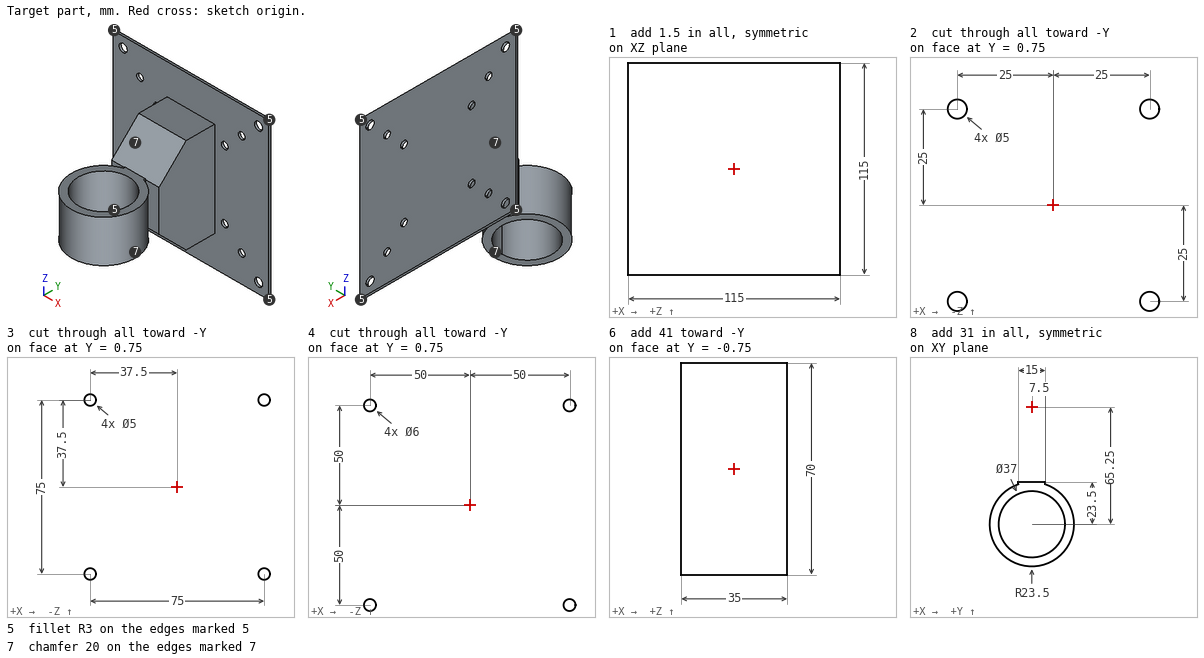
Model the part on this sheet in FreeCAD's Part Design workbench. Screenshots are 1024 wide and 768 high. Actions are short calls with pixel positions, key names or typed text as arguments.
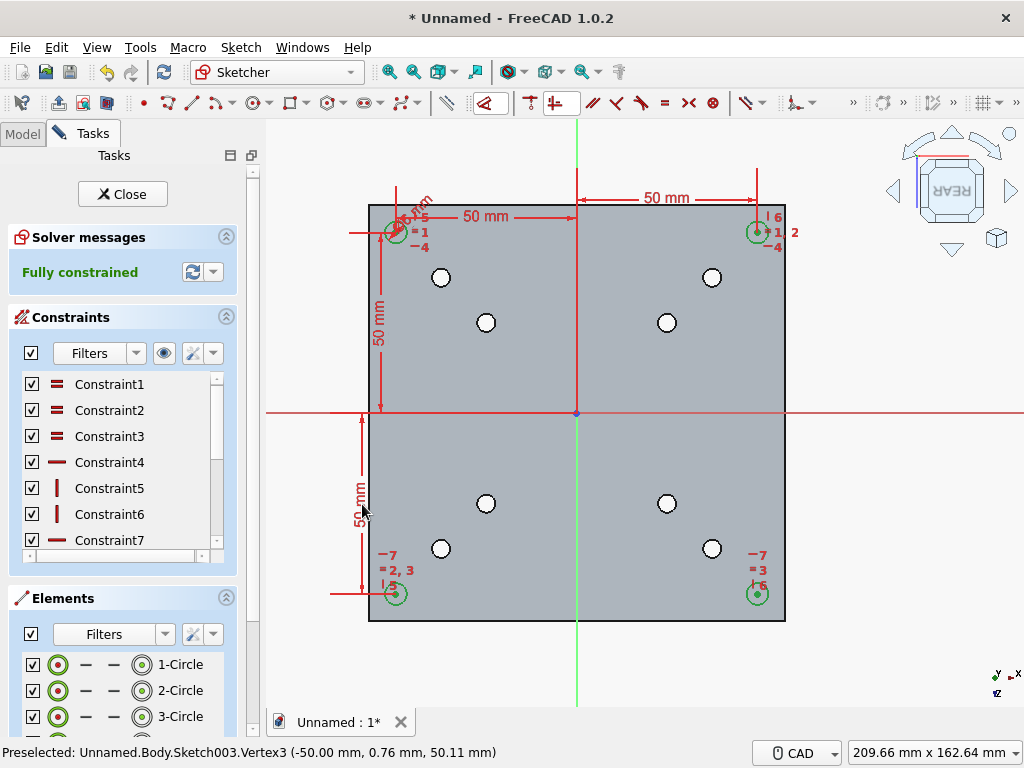
click(123, 194)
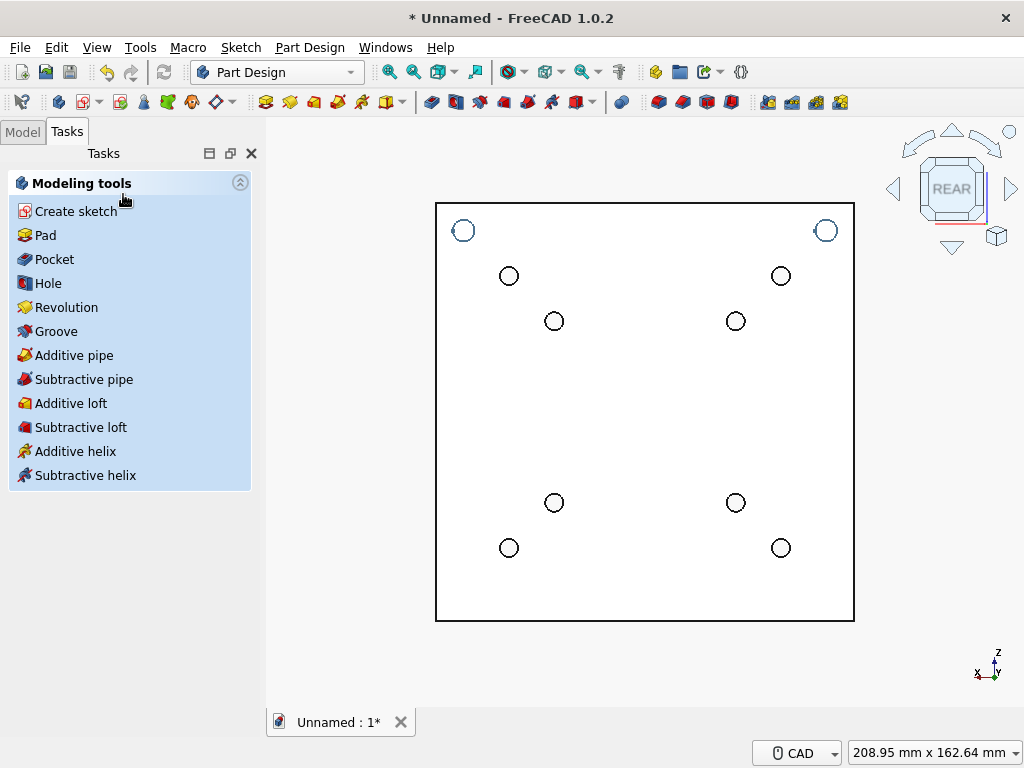
click(432, 102)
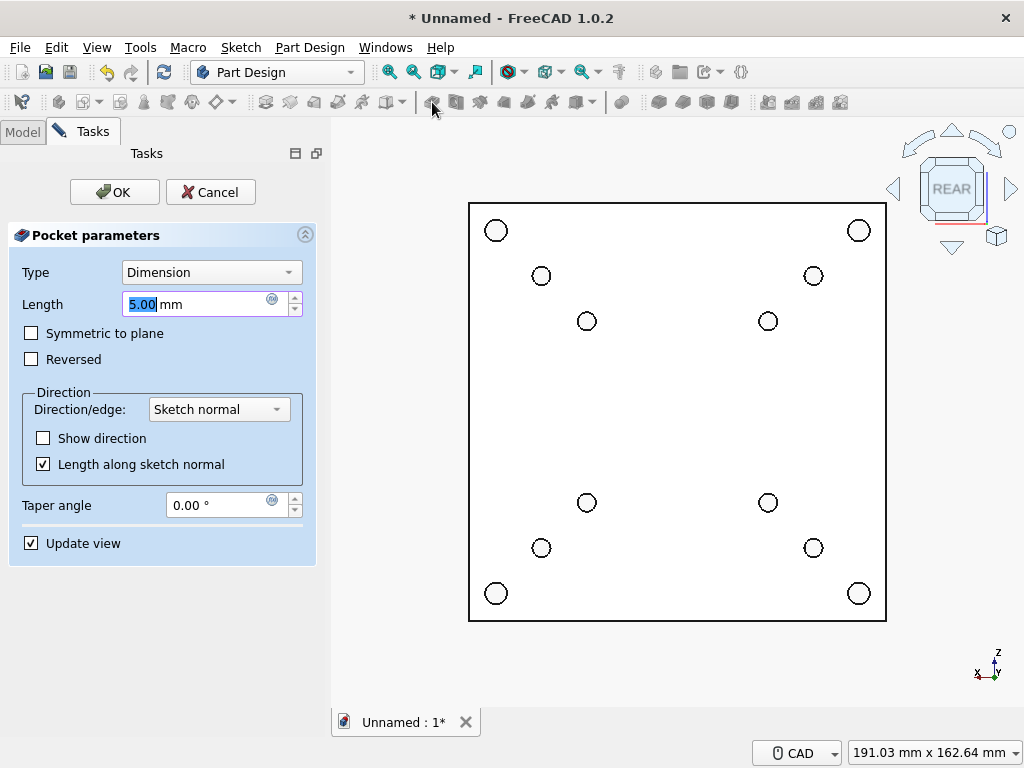
click(212, 272)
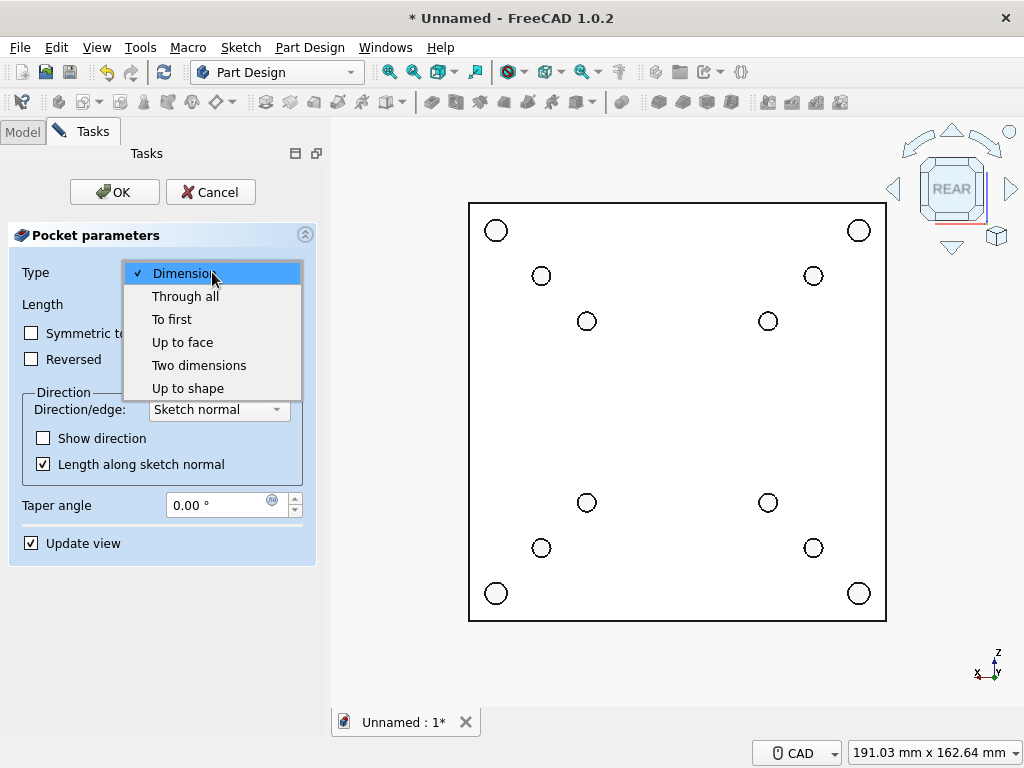
click(212, 296)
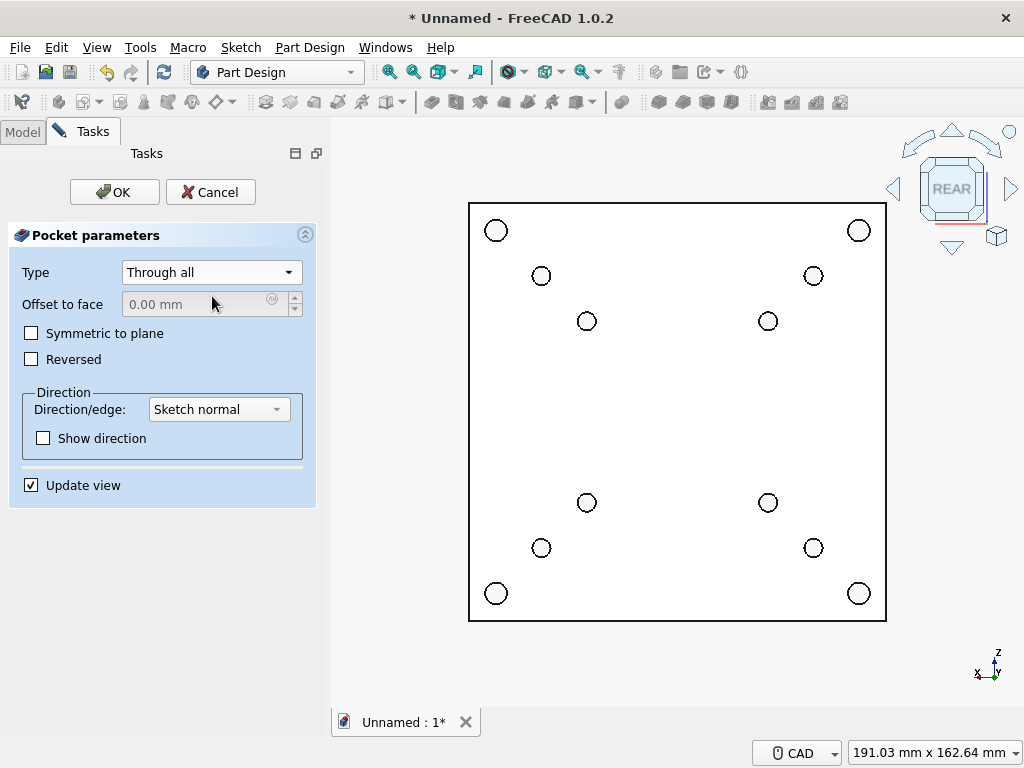
click(115, 192)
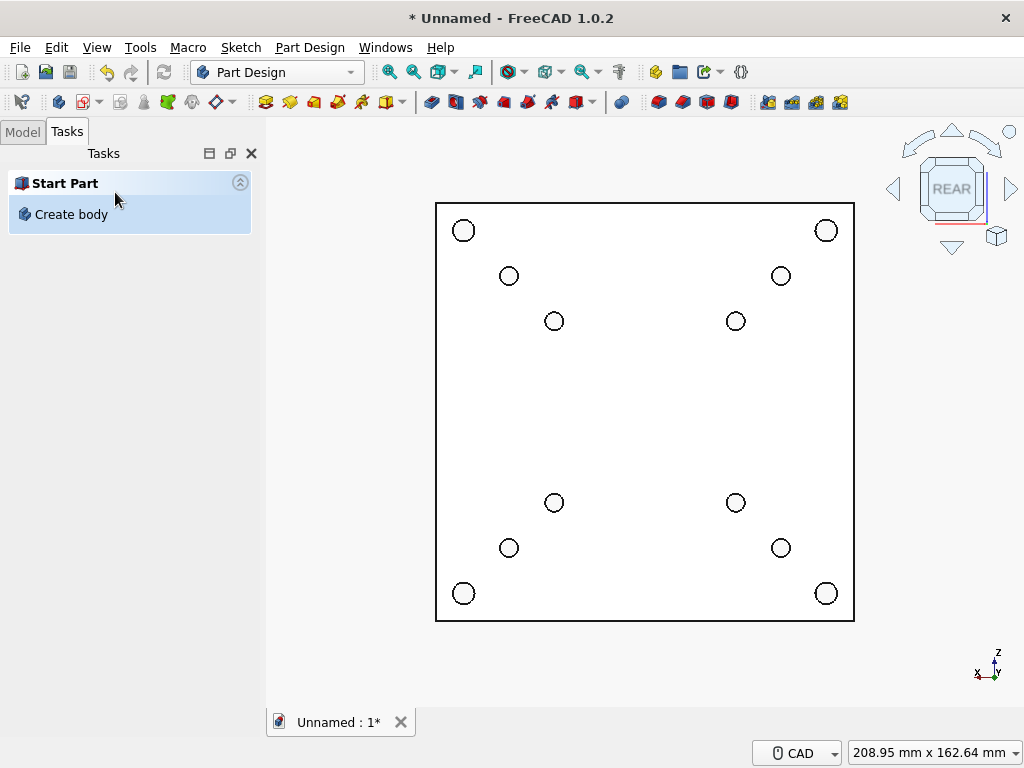
scroll(854, 620, up, 10)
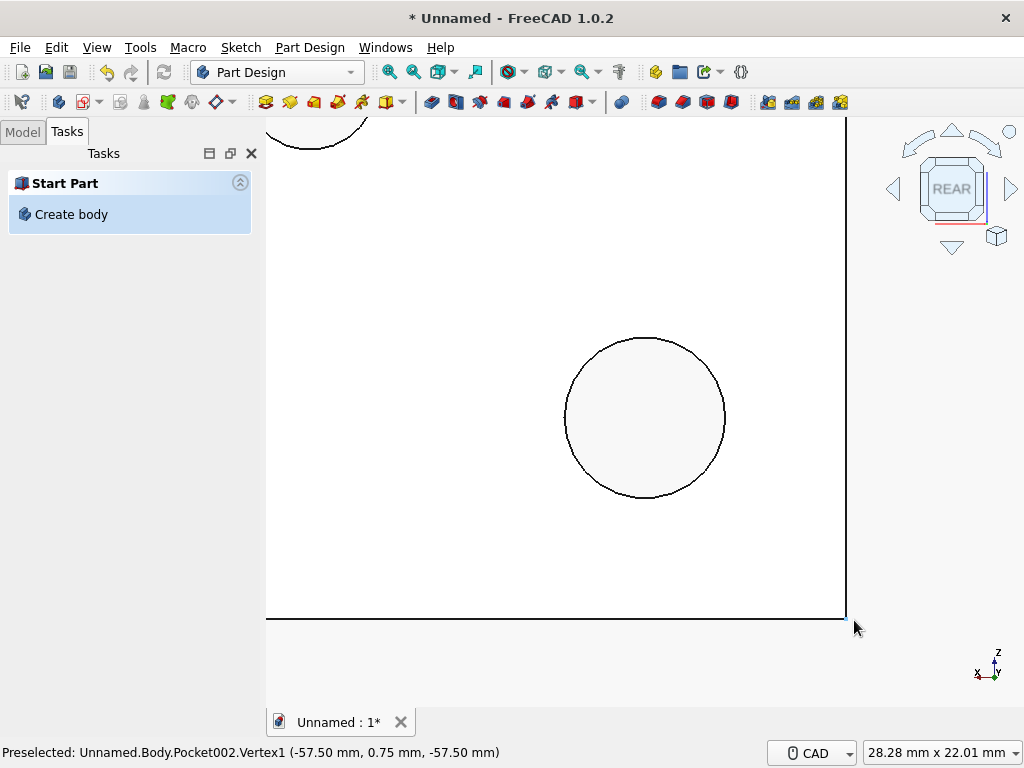
click(390, 72)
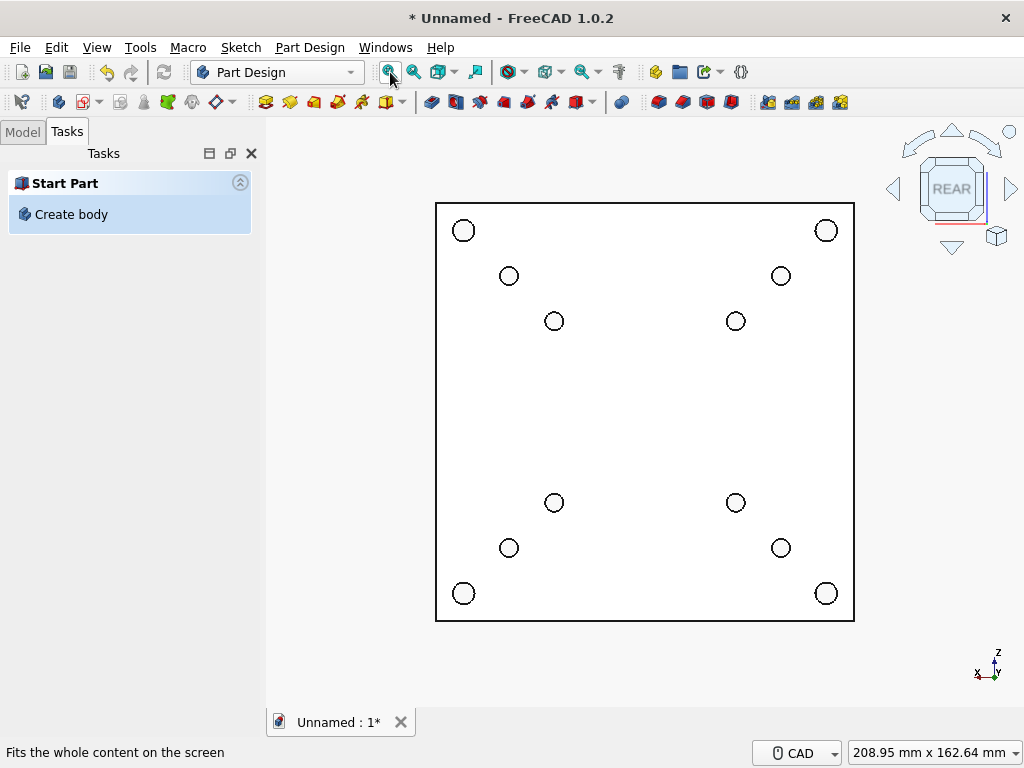
key(0)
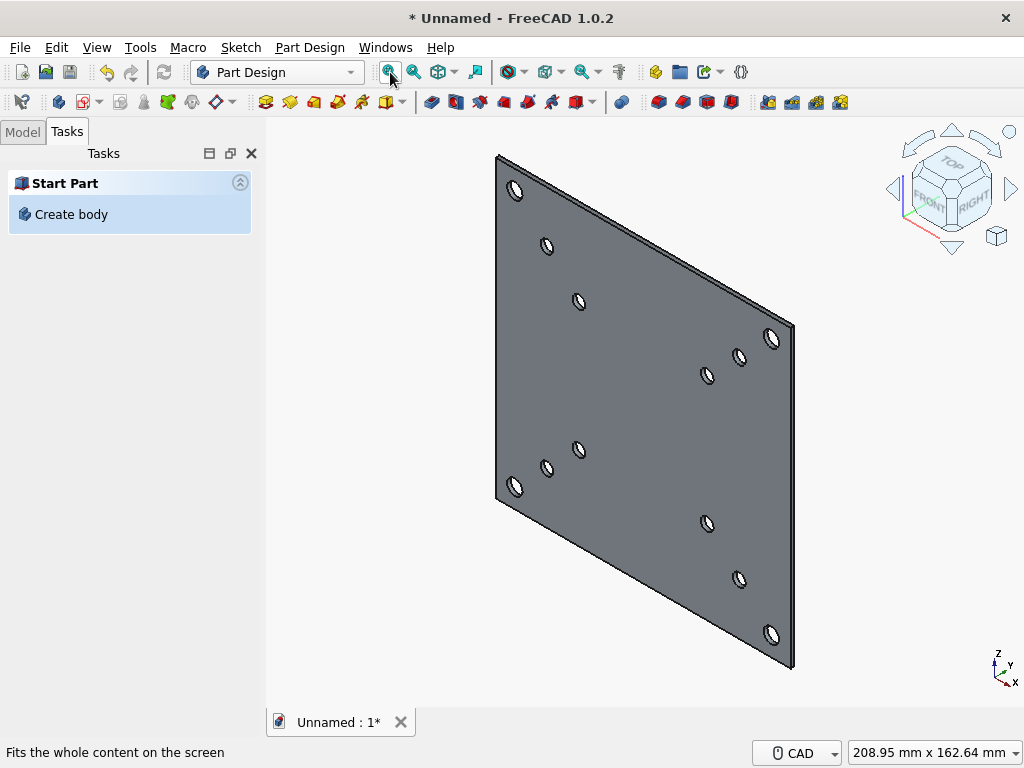
scroll(498, 496, up, 10)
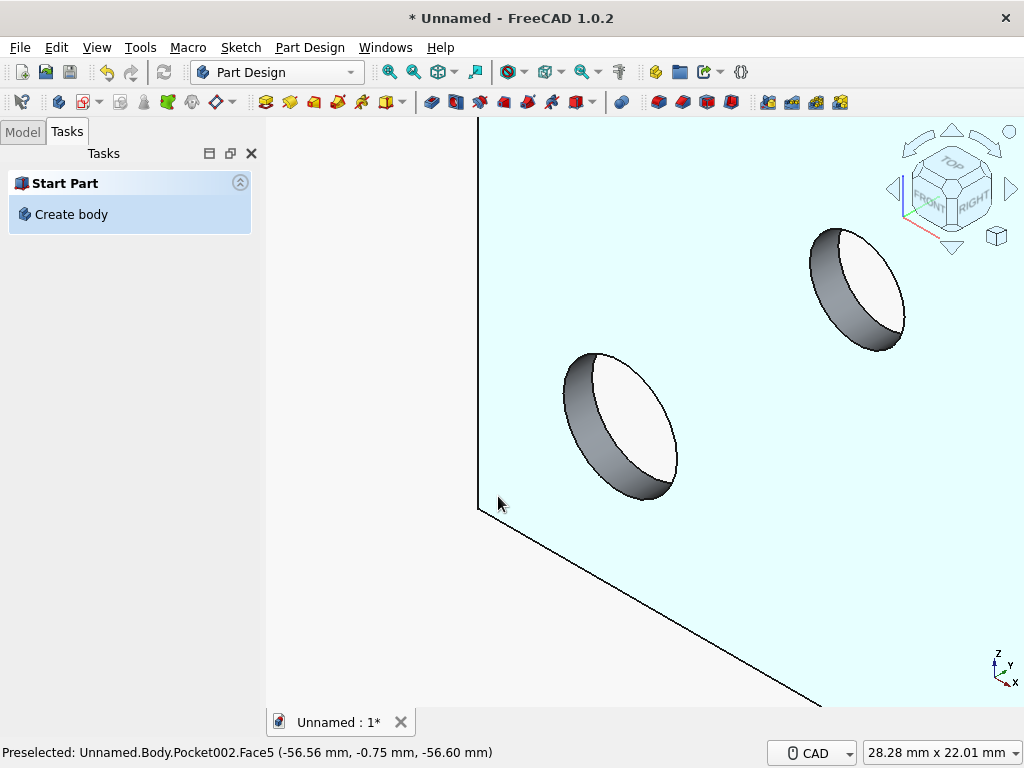
key(v)
key(f)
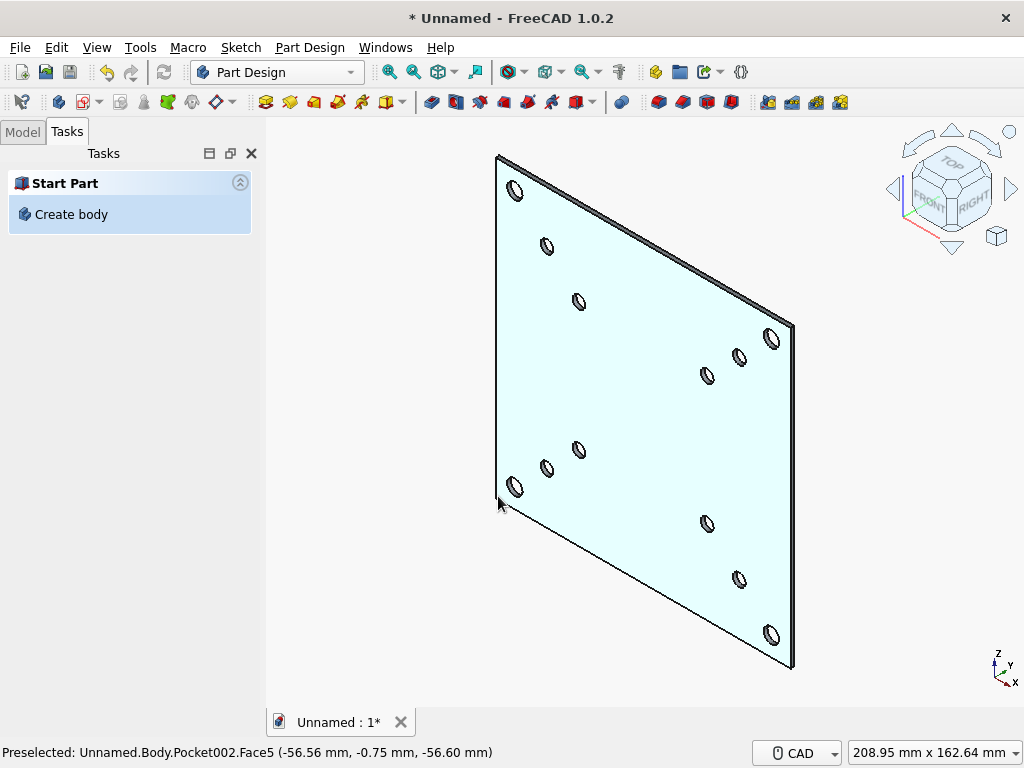
key(2)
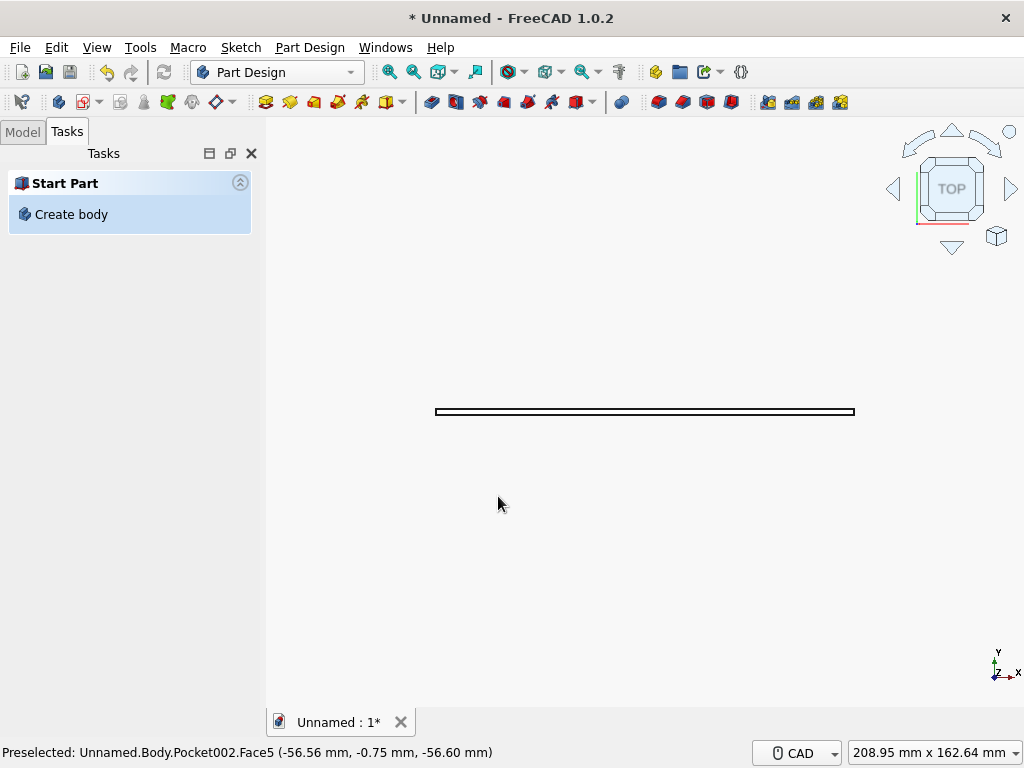
scroll(436, 411, up, 10)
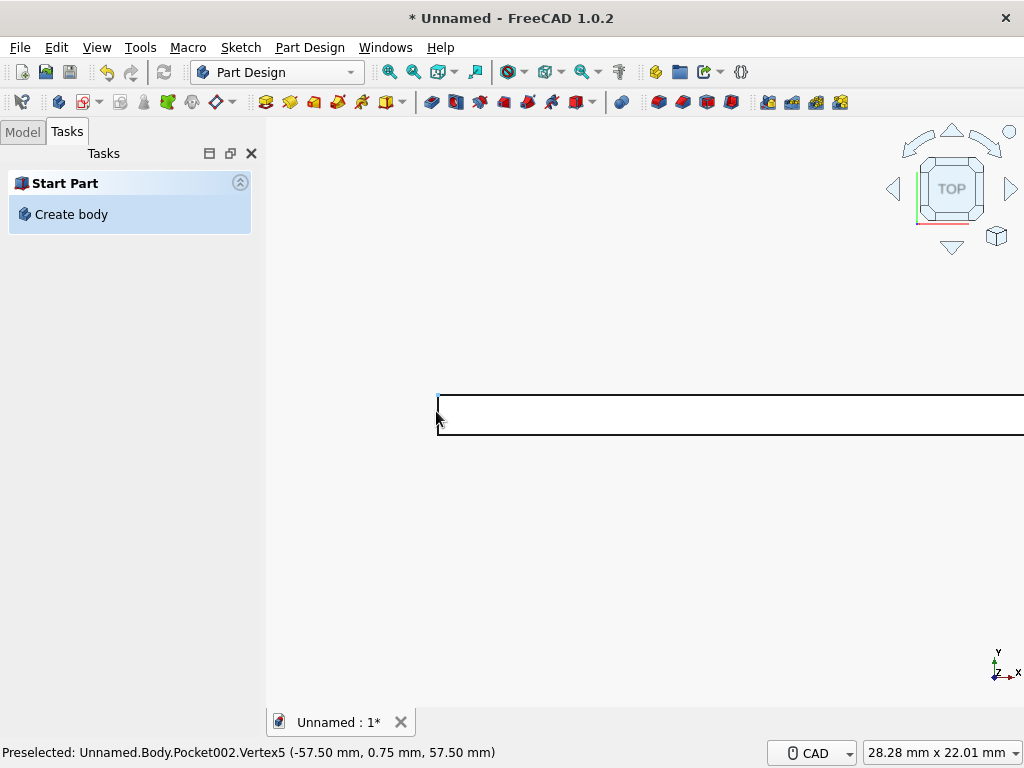
click(438, 414)